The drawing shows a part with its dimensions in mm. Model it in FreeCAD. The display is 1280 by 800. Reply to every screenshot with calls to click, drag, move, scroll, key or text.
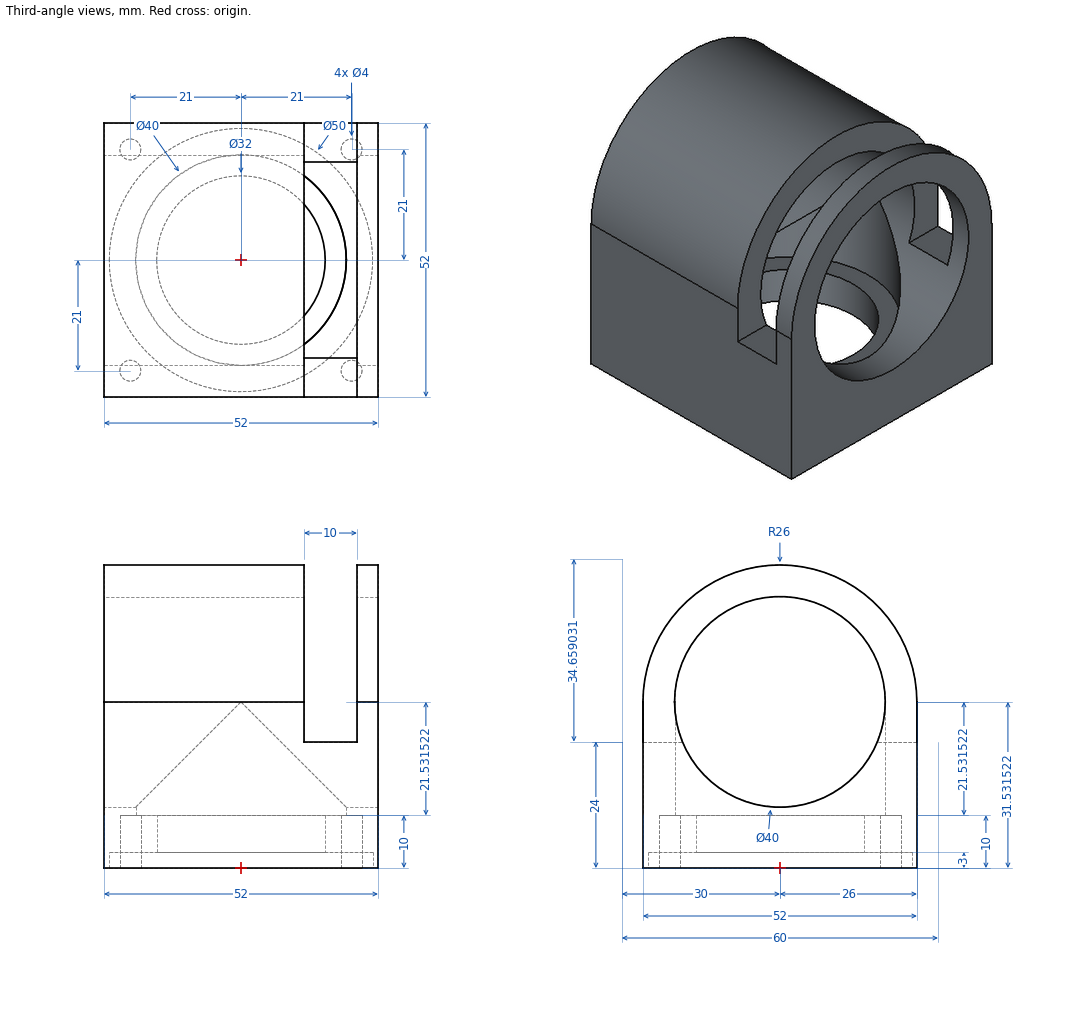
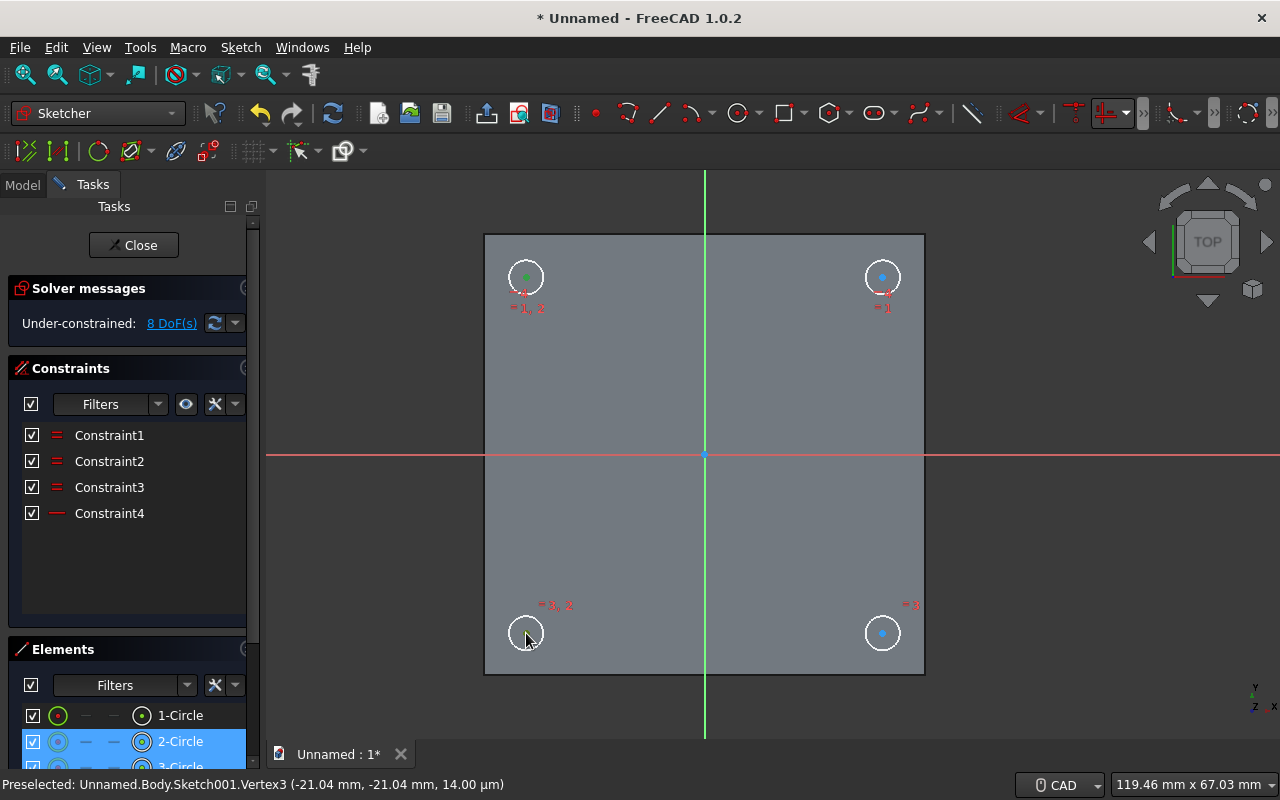
key(v)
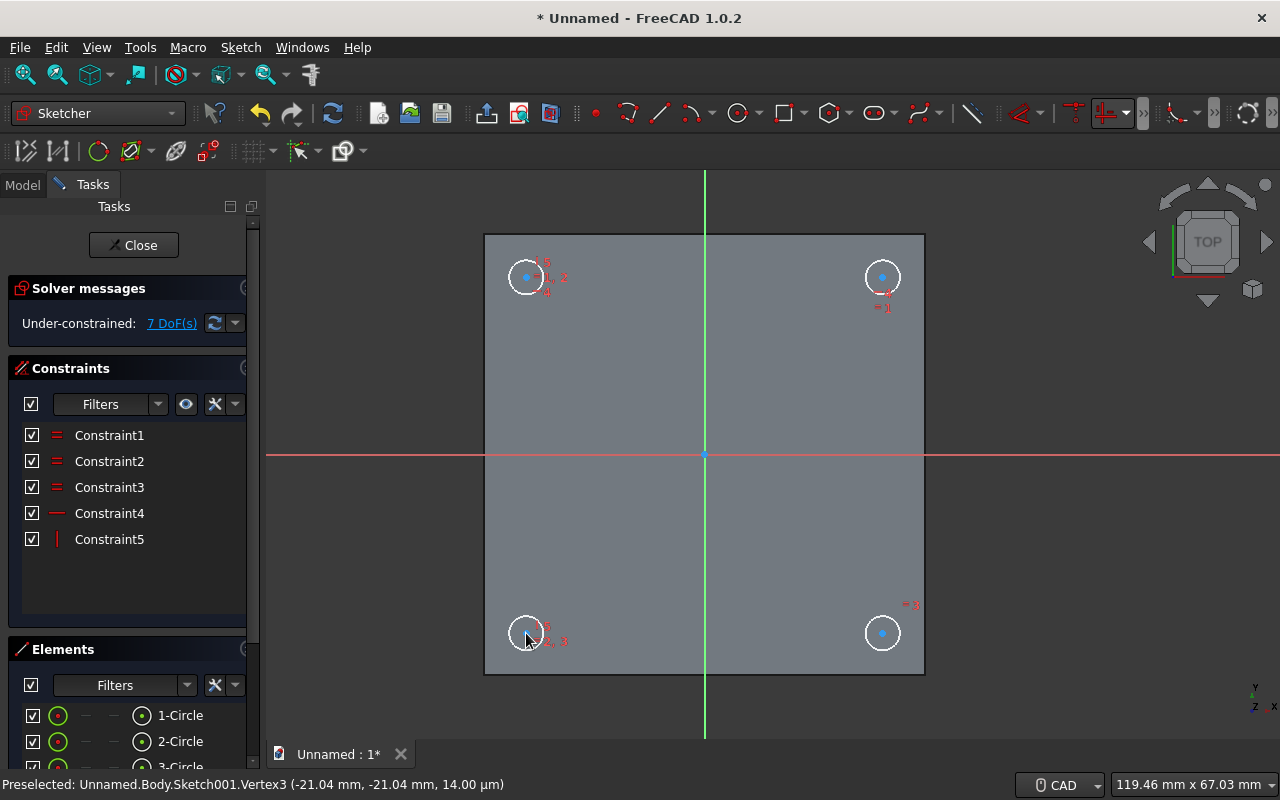
click(883, 277)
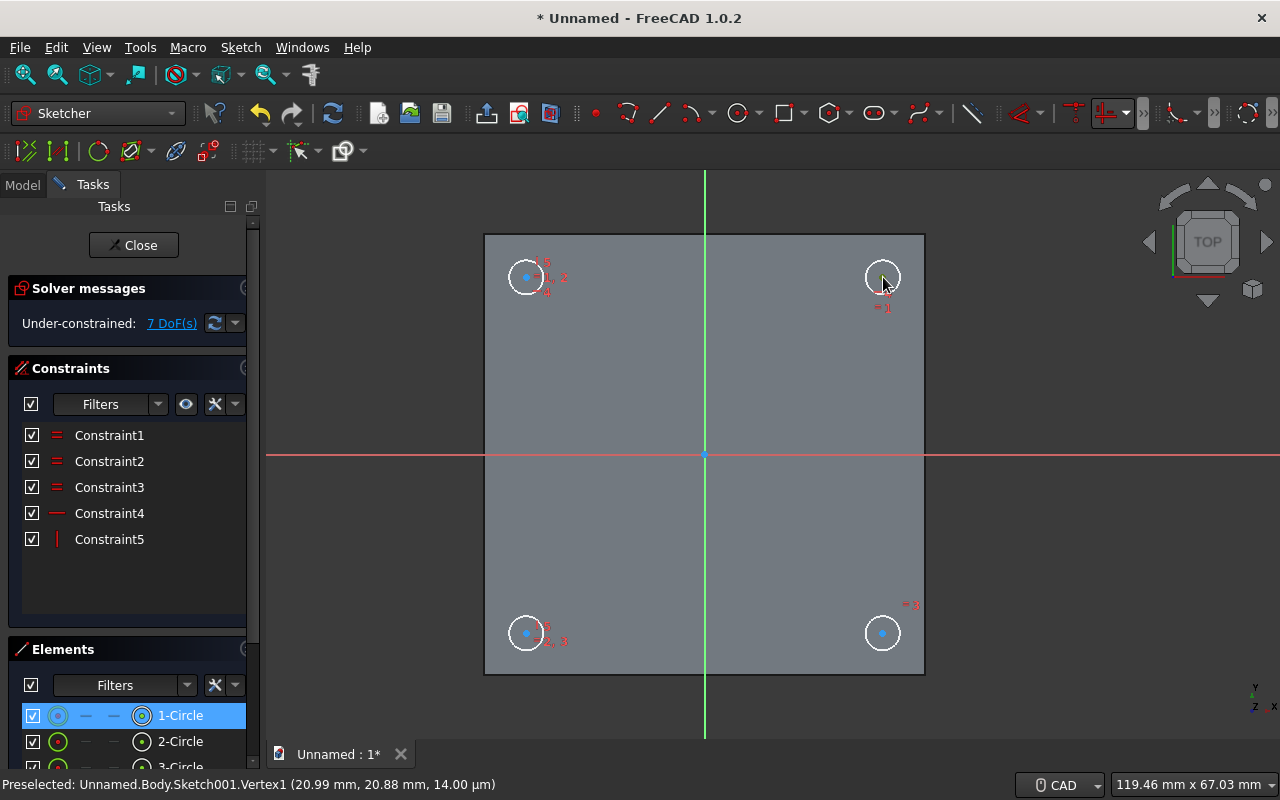
click(883, 633)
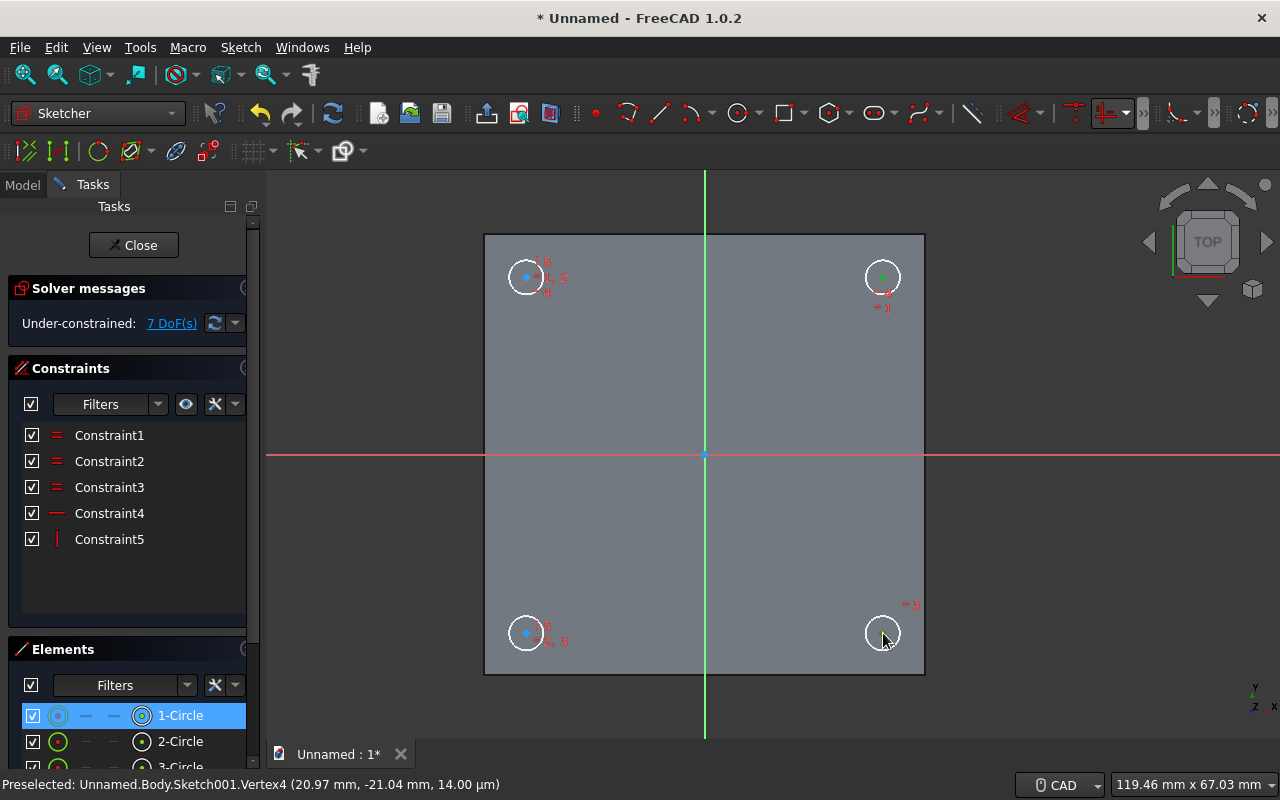
click(1128, 114)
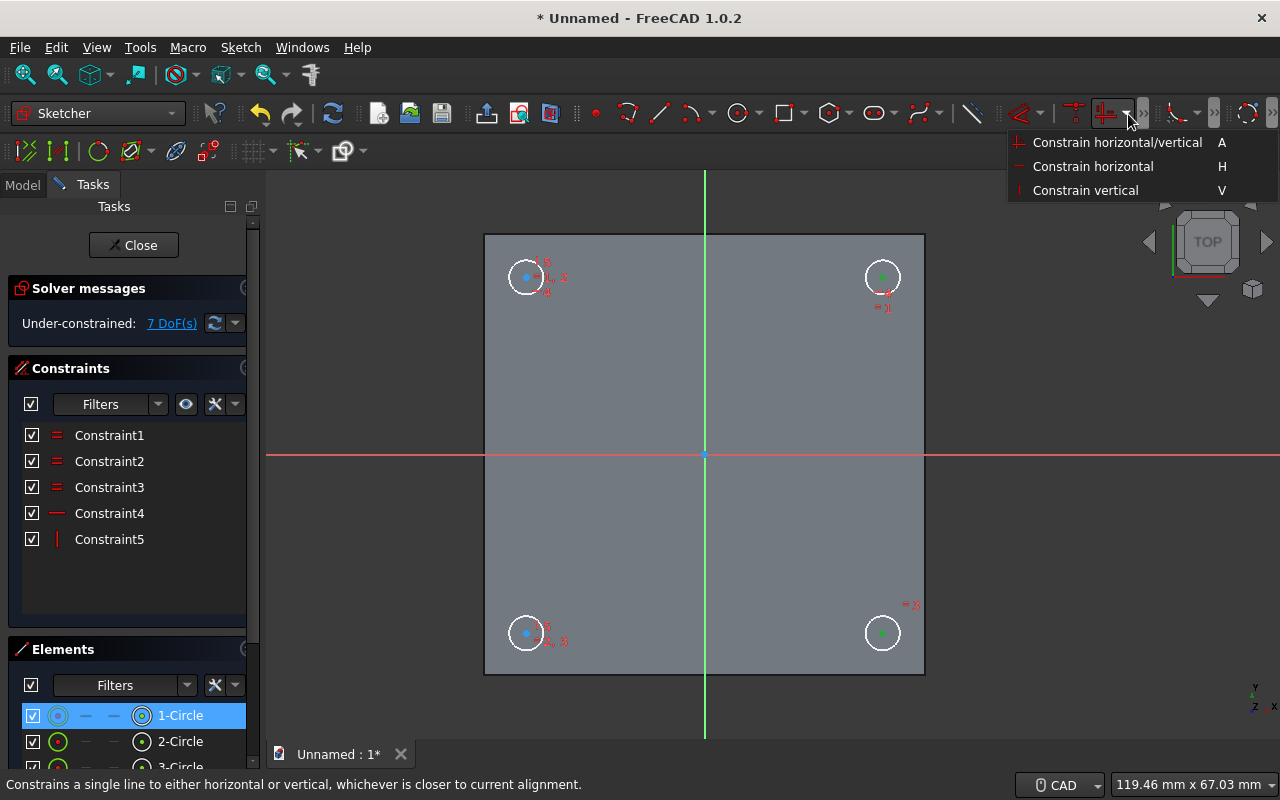
click(1143, 190)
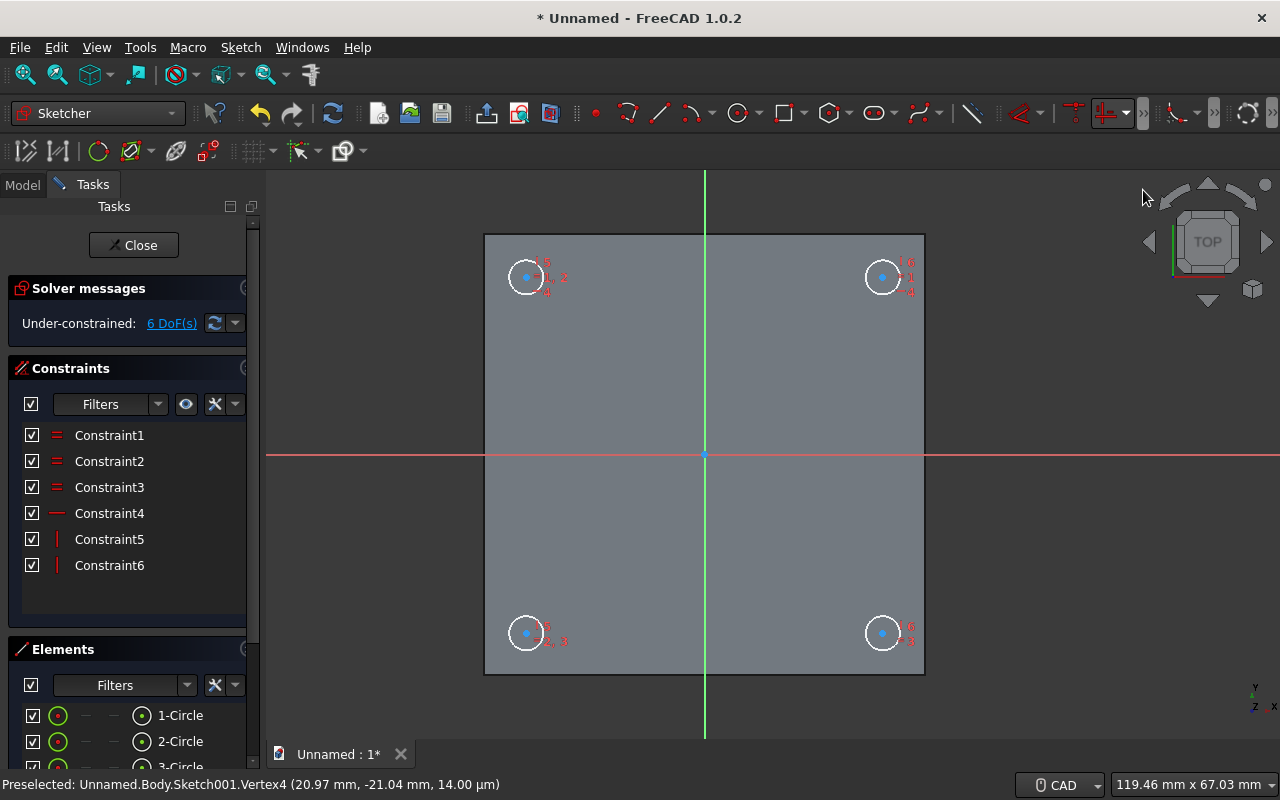
click(526, 633)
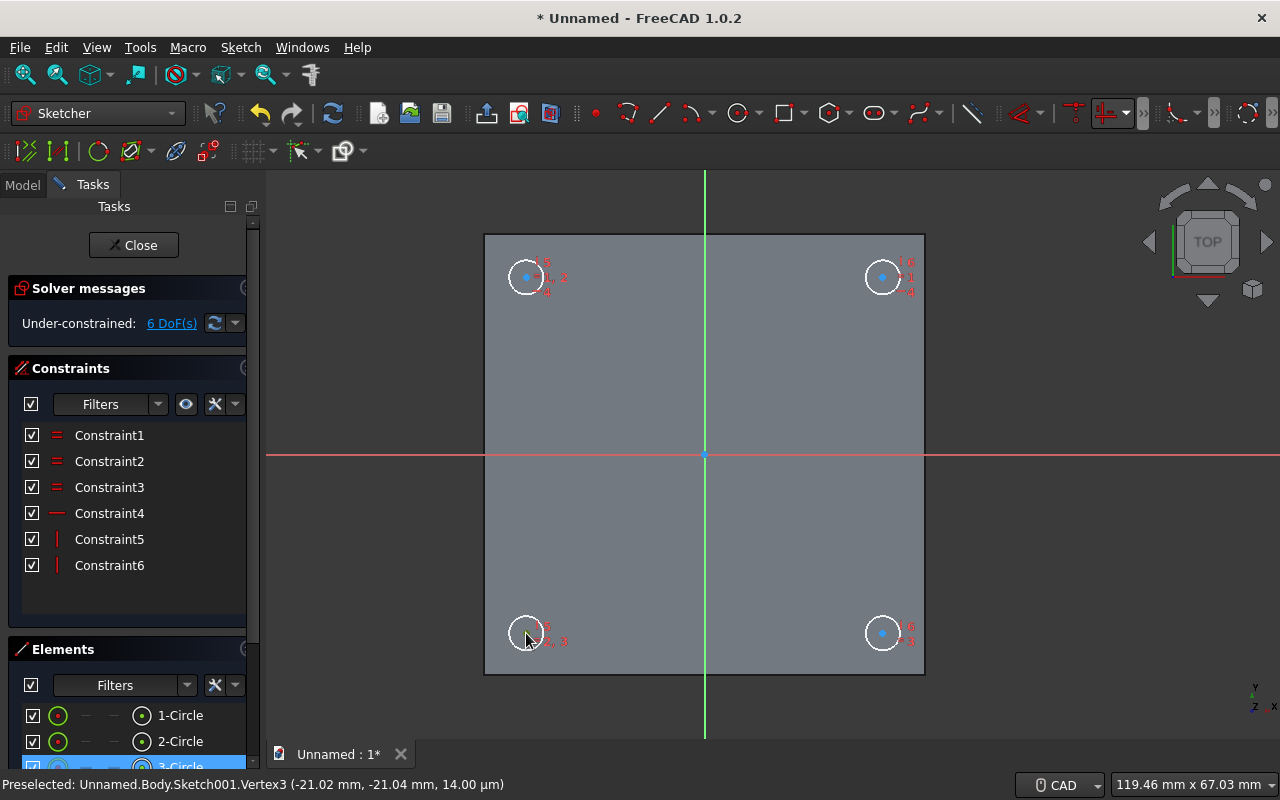
click(883, 633)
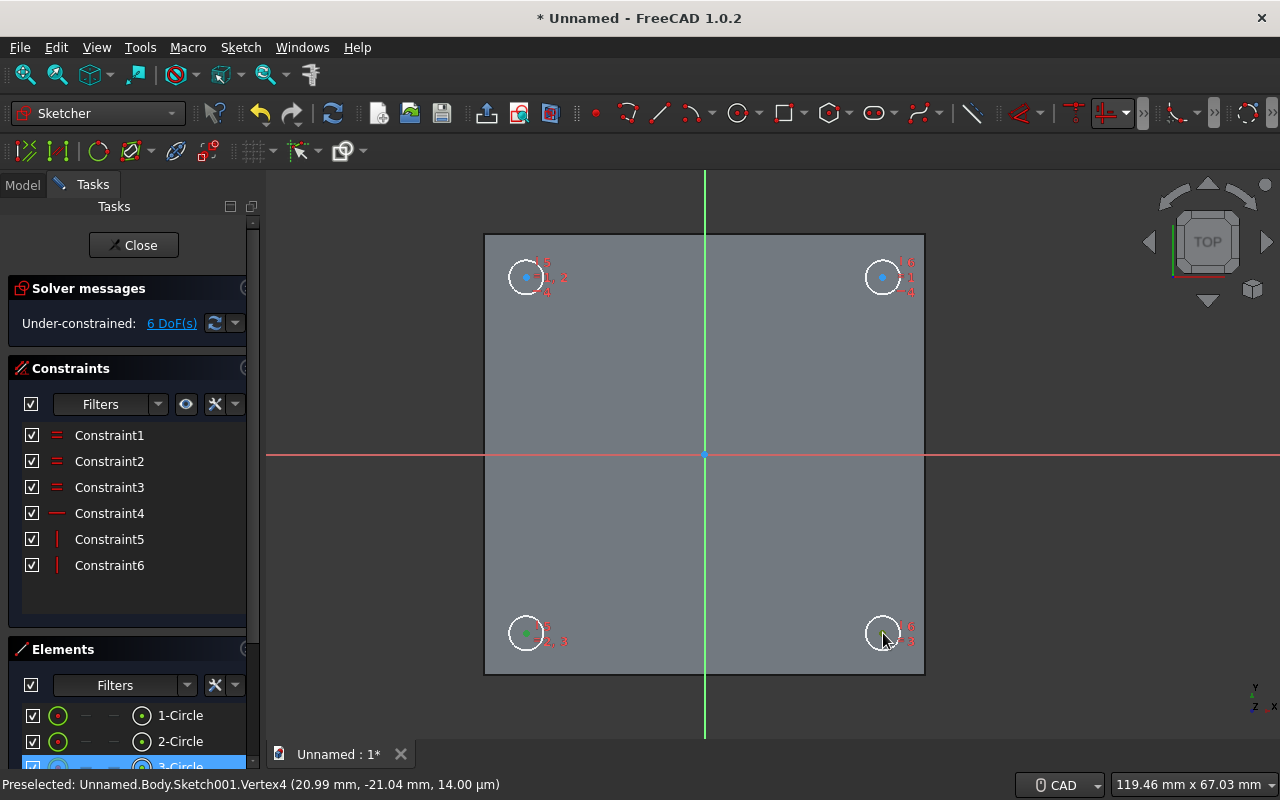
key(h)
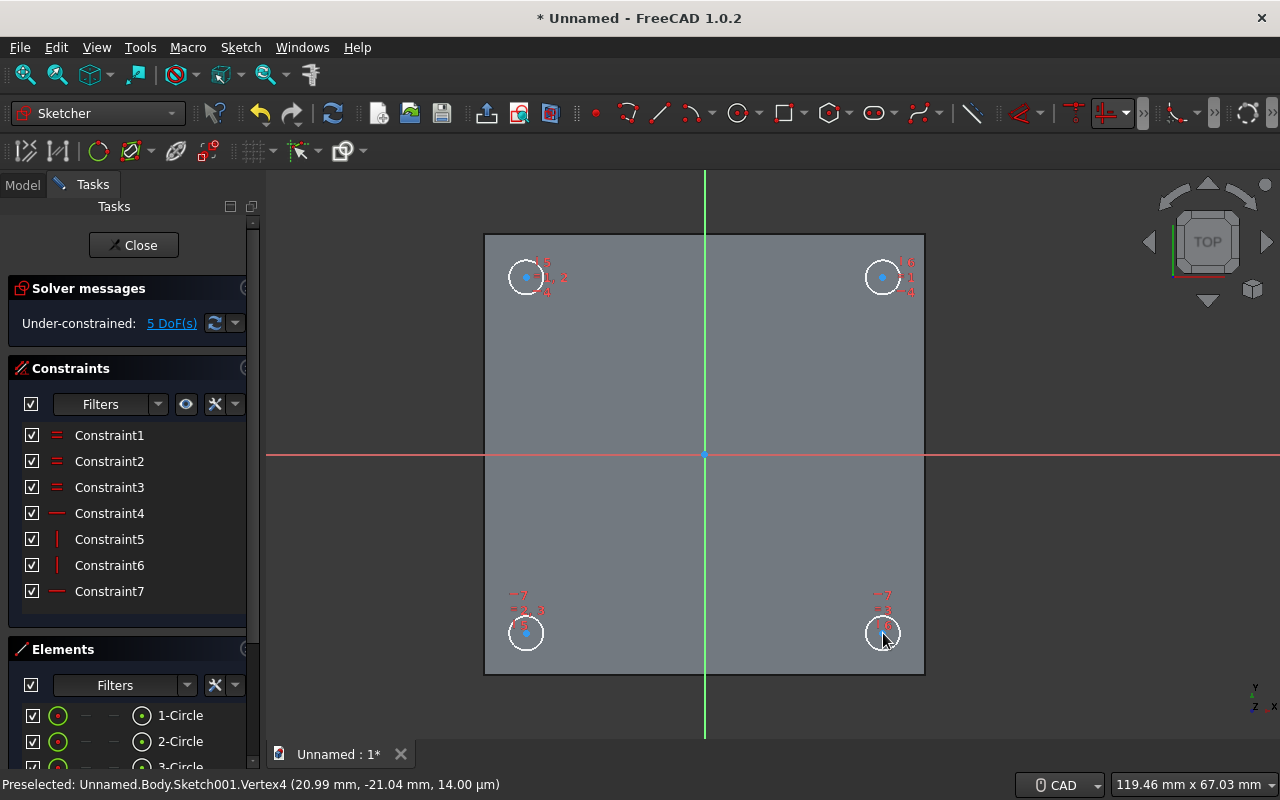
click(1020, 114)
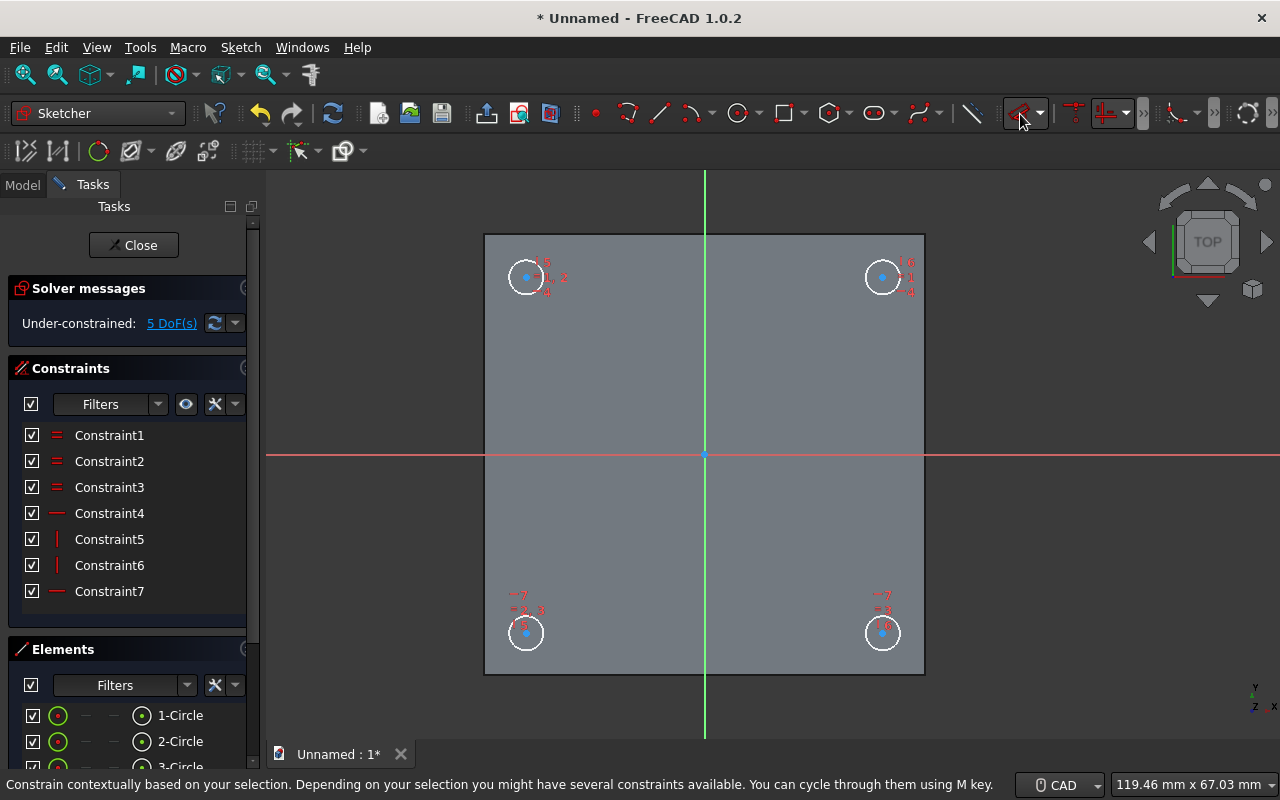
click(895, 265)
click(917, 242)